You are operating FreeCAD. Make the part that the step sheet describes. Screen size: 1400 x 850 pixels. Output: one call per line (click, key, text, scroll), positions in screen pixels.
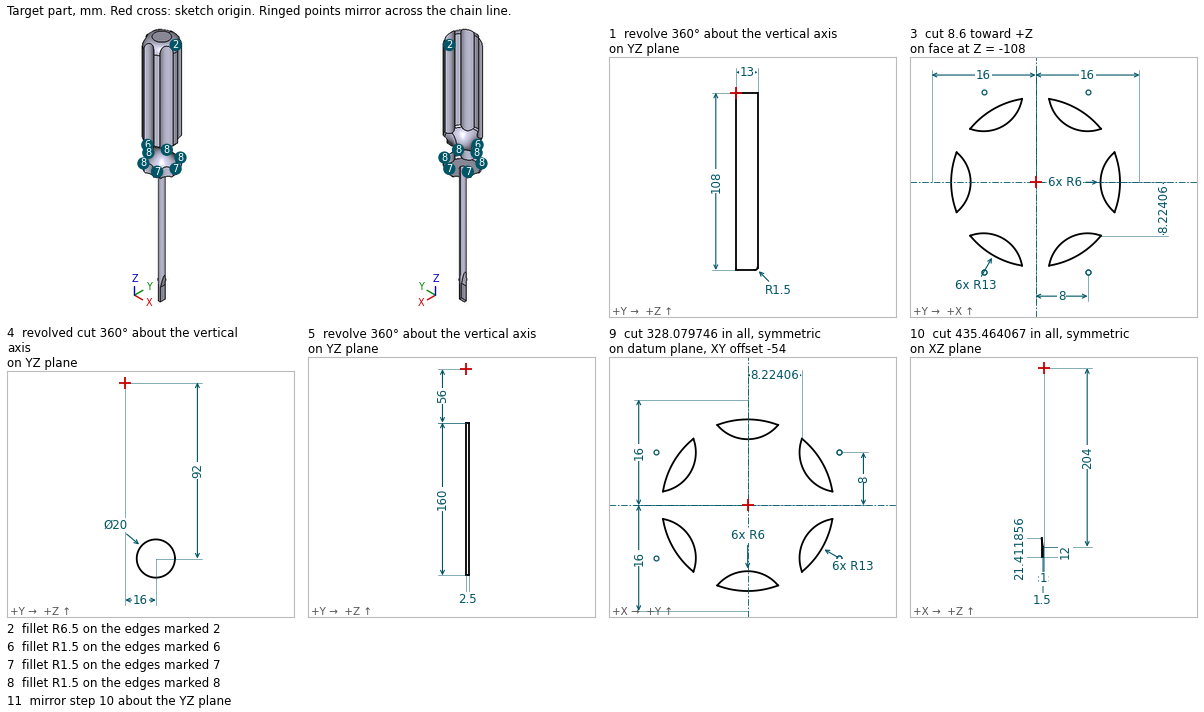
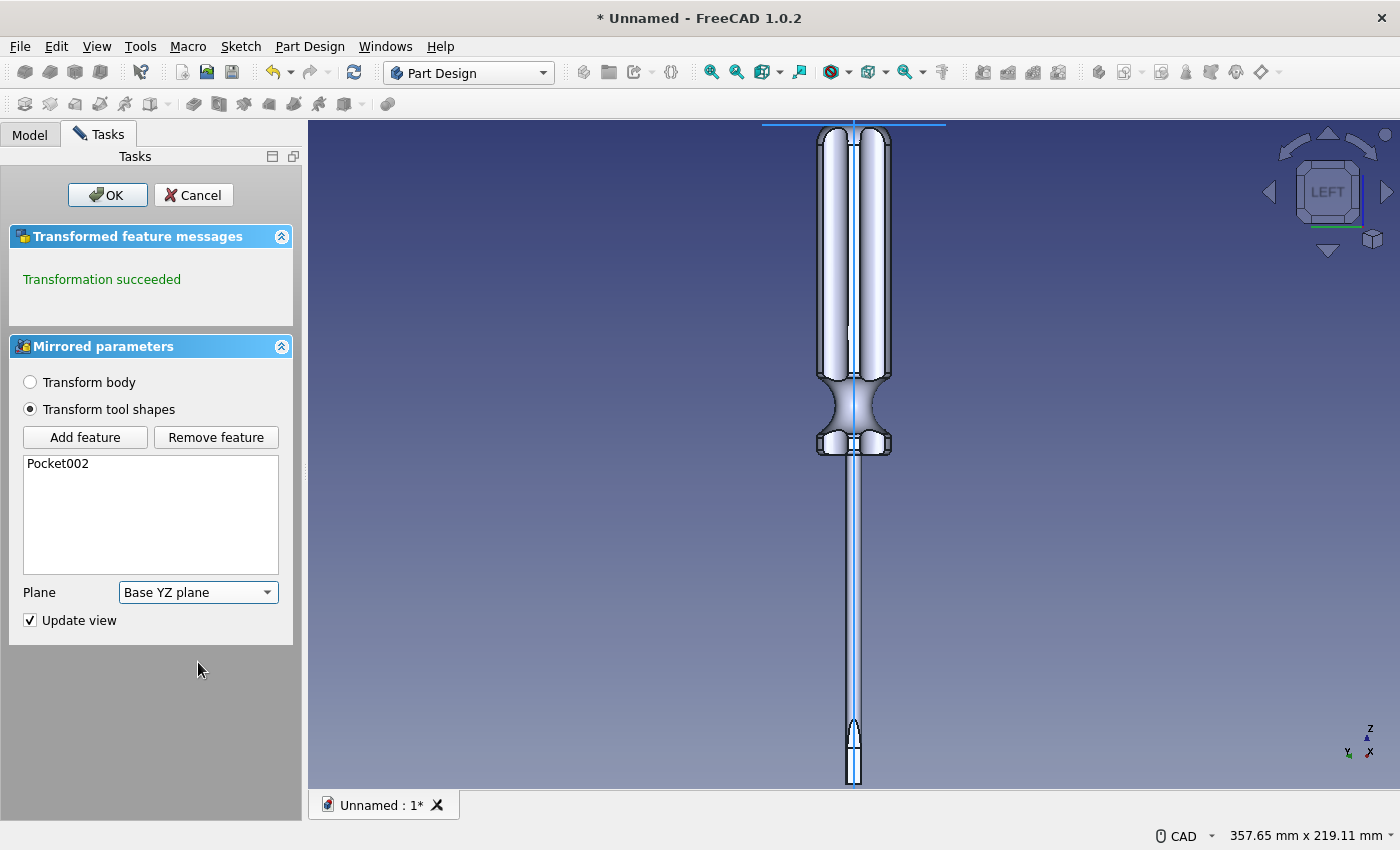
click(108, 195)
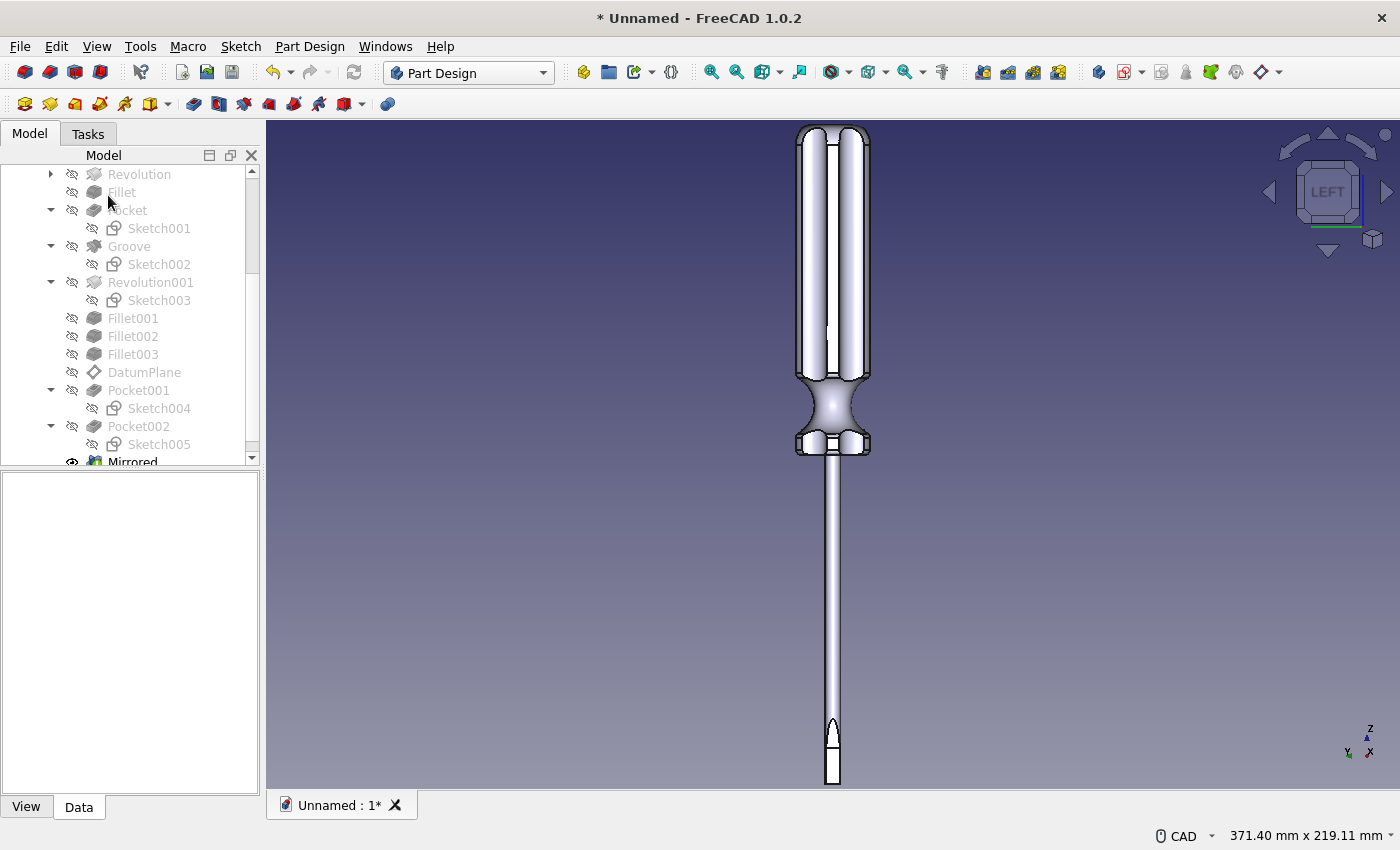
key(0)